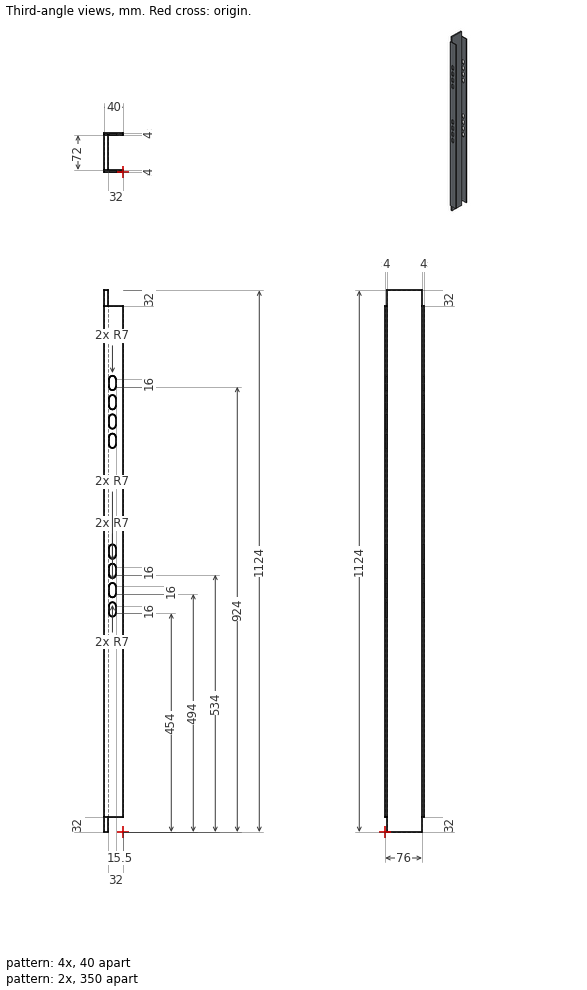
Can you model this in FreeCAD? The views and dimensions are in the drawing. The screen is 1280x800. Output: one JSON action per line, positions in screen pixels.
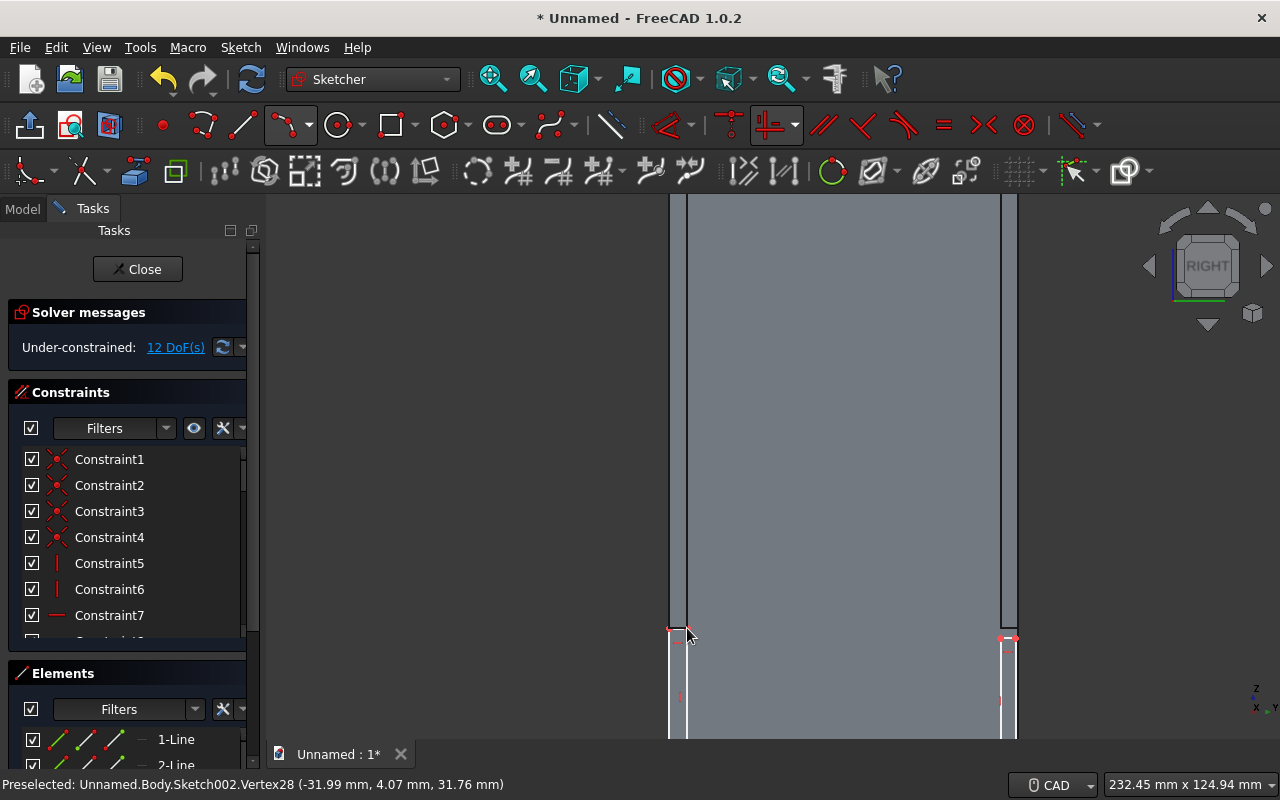
{"action": "left_click", "coordinate": [666, 126]}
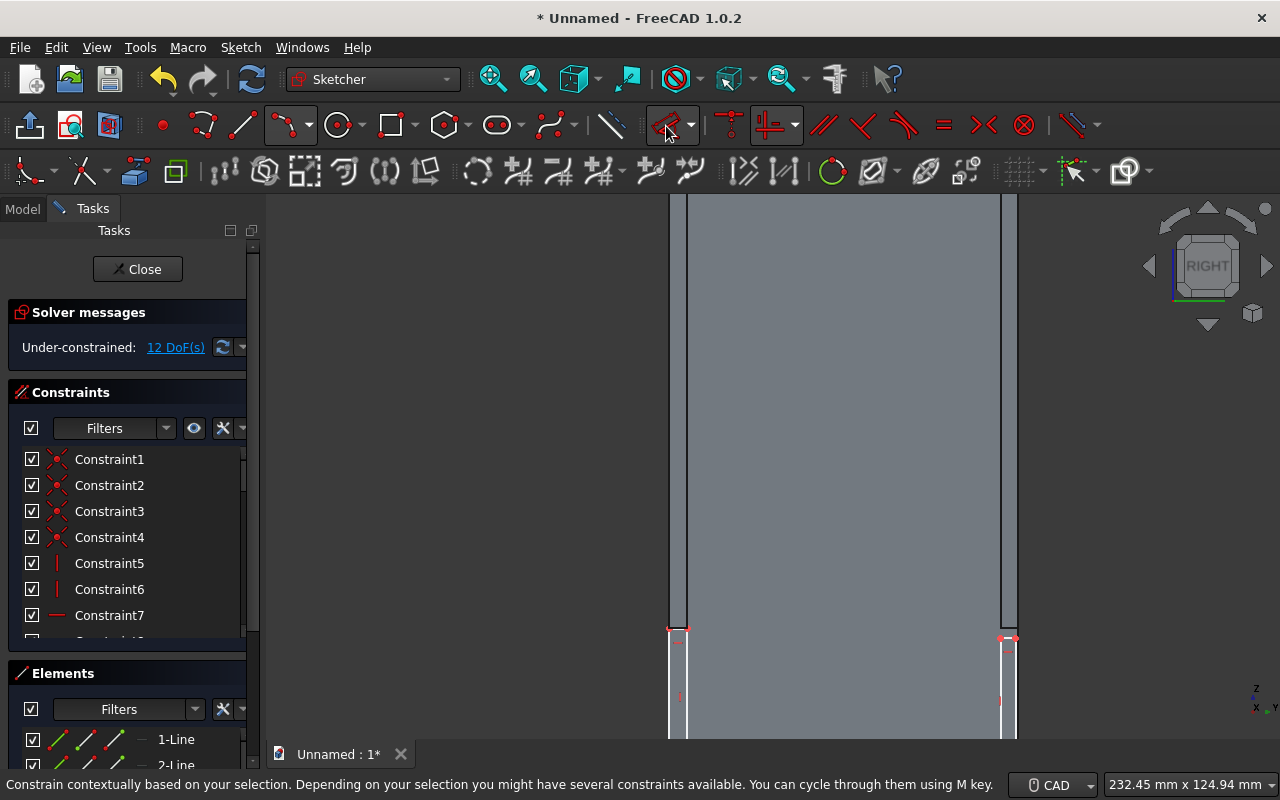
{"action": "scroll", "coordinate": [693, 639], "scroll_direction": "down", "scroll_amount": 13}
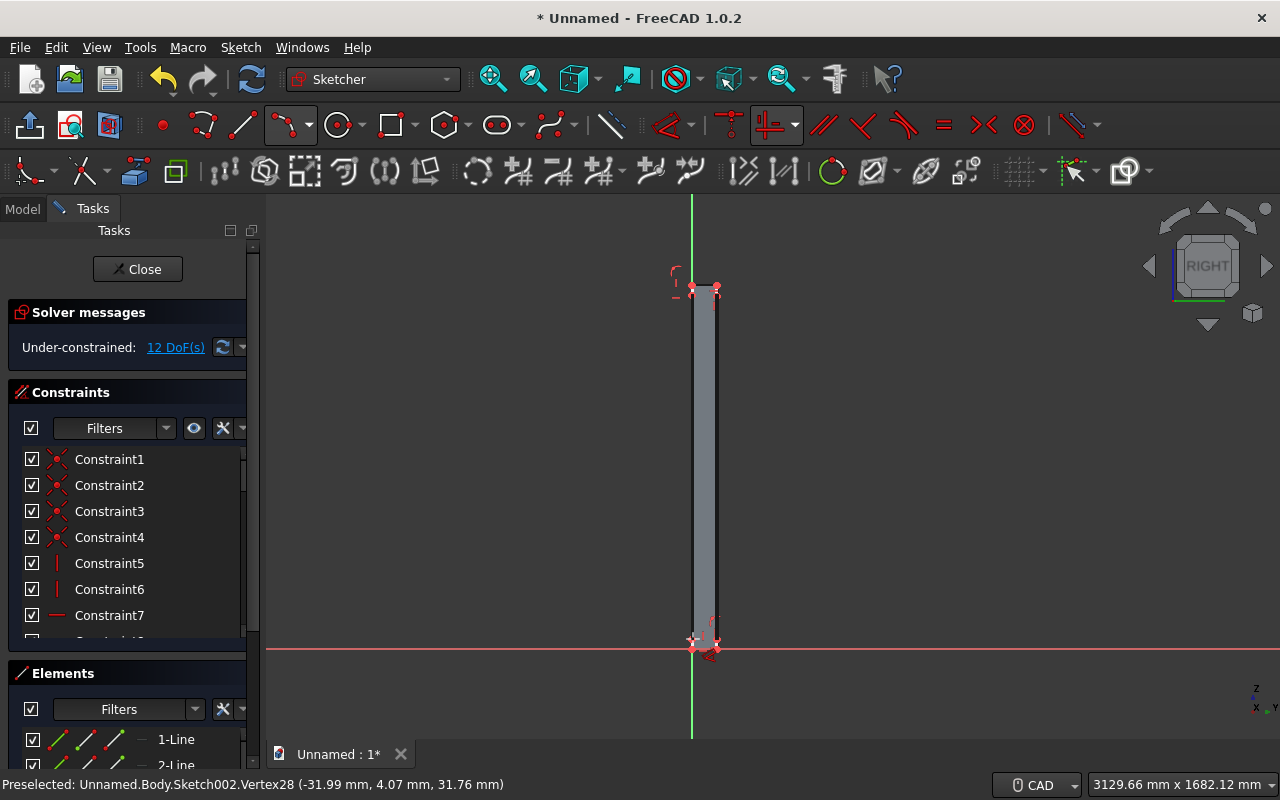
{"action": "scroll", "coordinate": [717, 297], "scroll_direction": "up", "scroll_amount": 18}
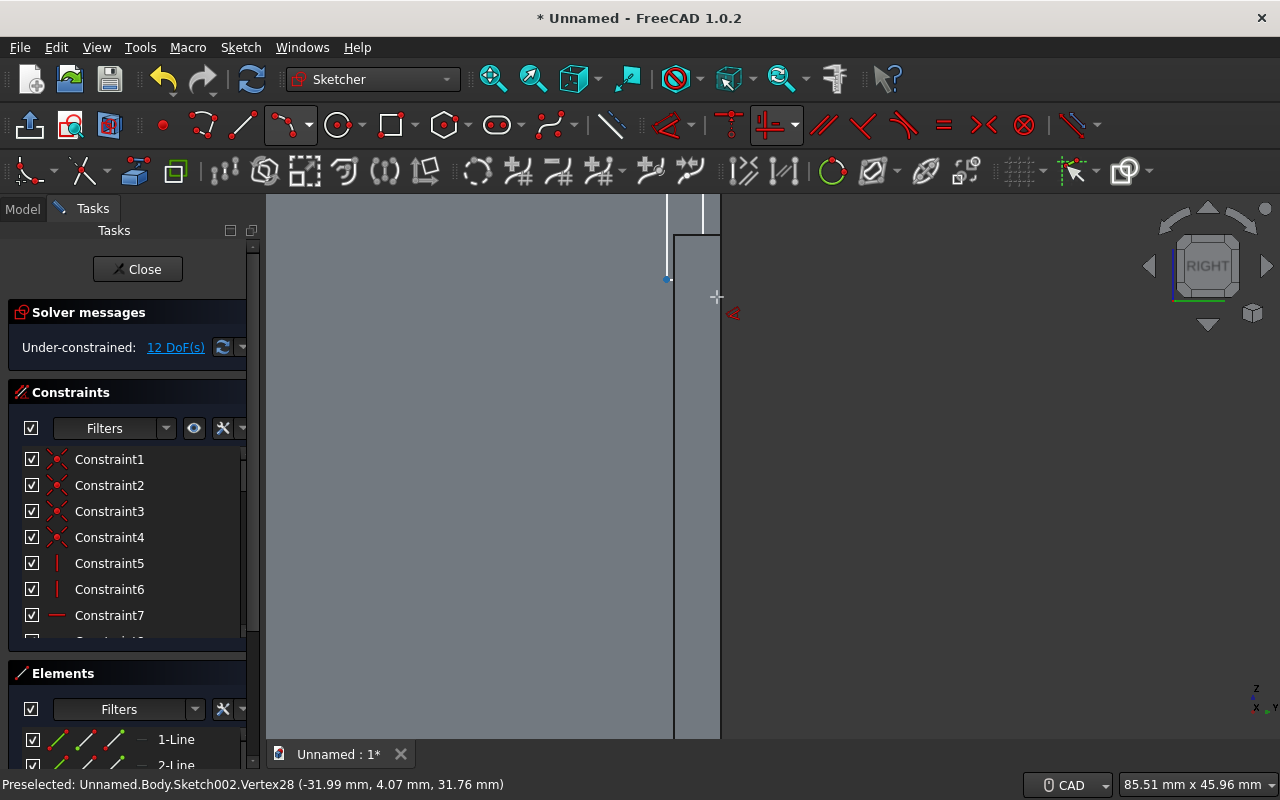
{"action": "left_click", "coordinate": [685, 280]}
{"action": "left_click", "coordinate": [685, 246]}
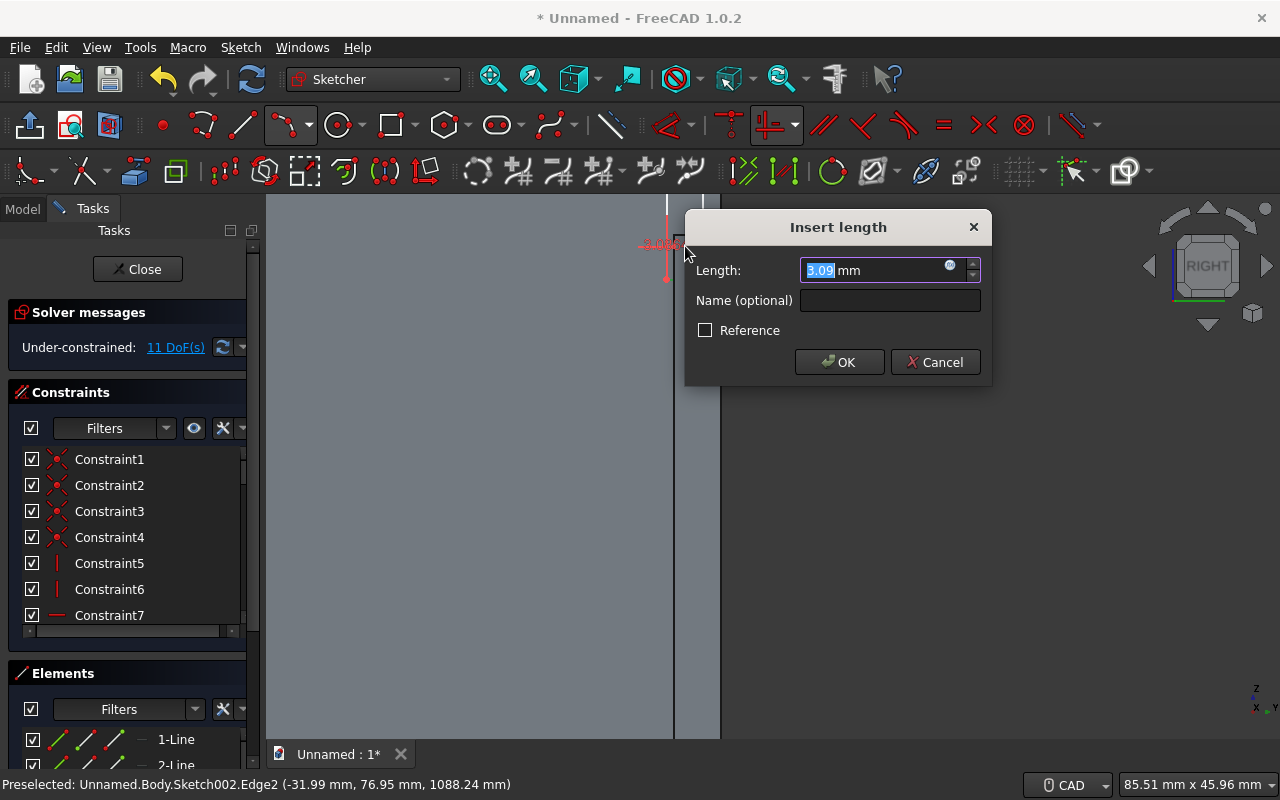
{"action": "type", "text": "4"}
{"action": "key", "text": "Return"}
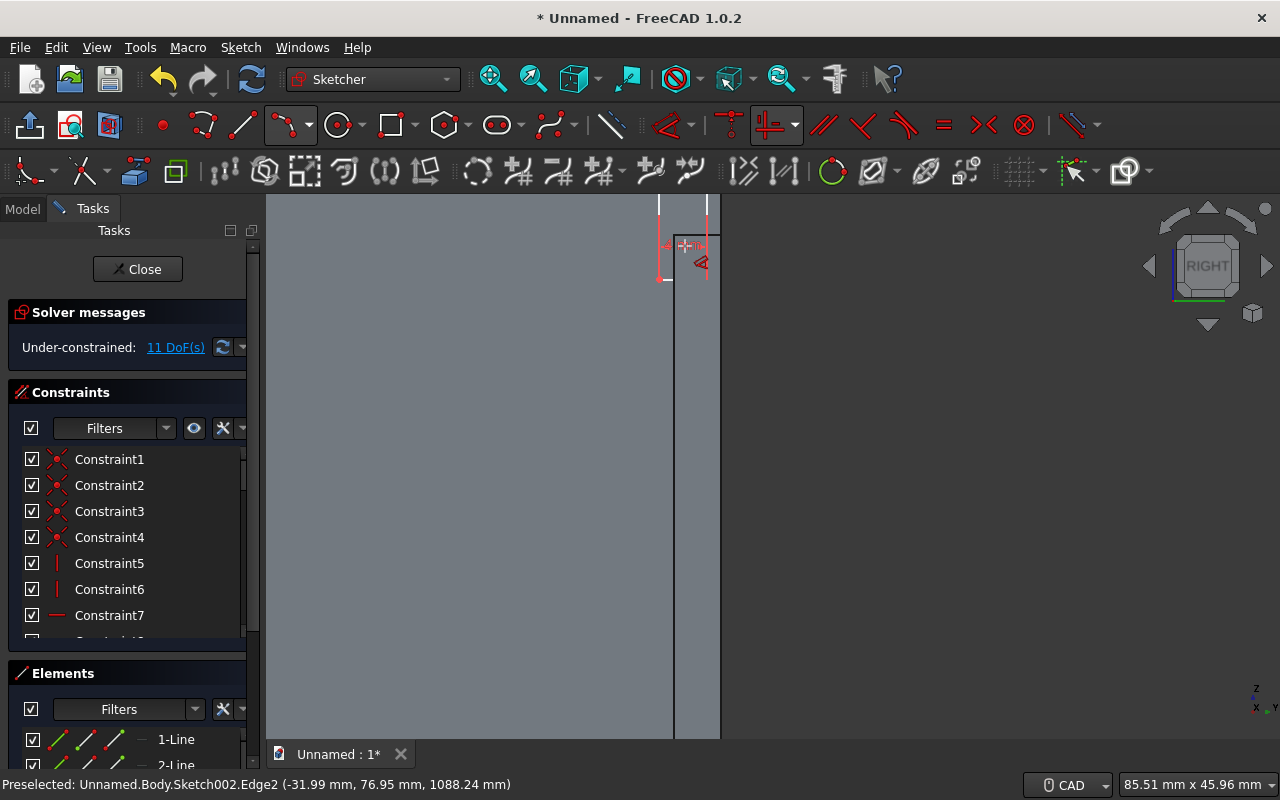
{"action": "scroll", "coordinate": [717, 296], "scroll_direction": "down", "scroll_amount": 18}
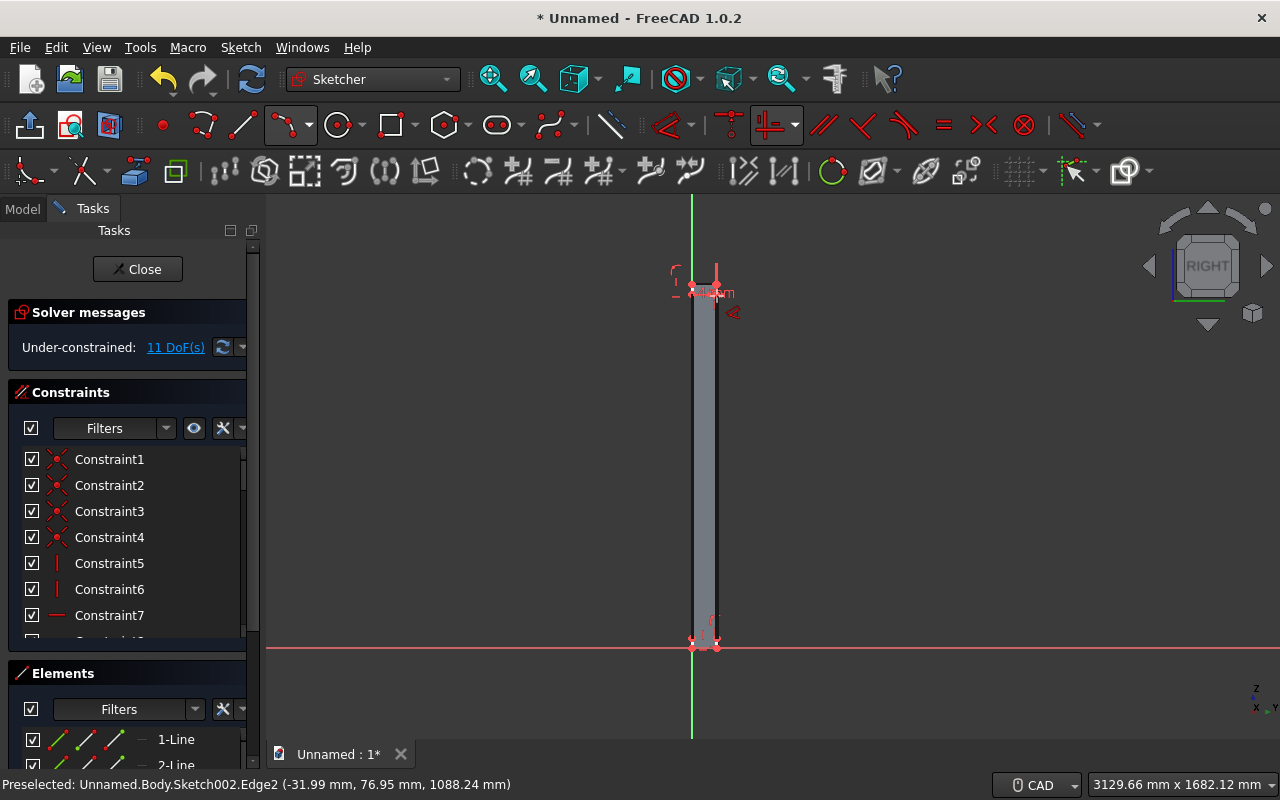
{"action": "scroll", "coordinate": [692, 295], "scroll_direction": "up", "scroll_amount": 18}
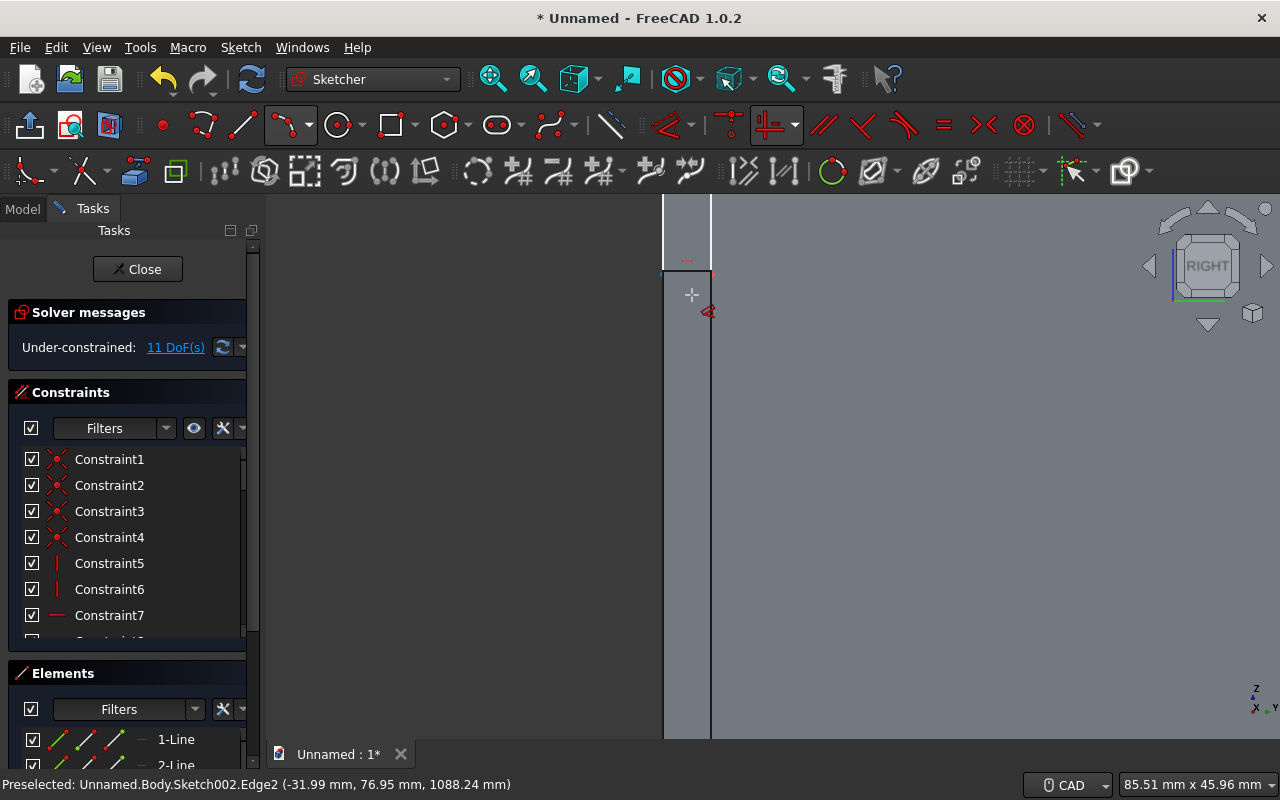
{"action": "left_click", "coordinate": [678, 274]}
{"action": "left_click", "coordinate": [687, 240]}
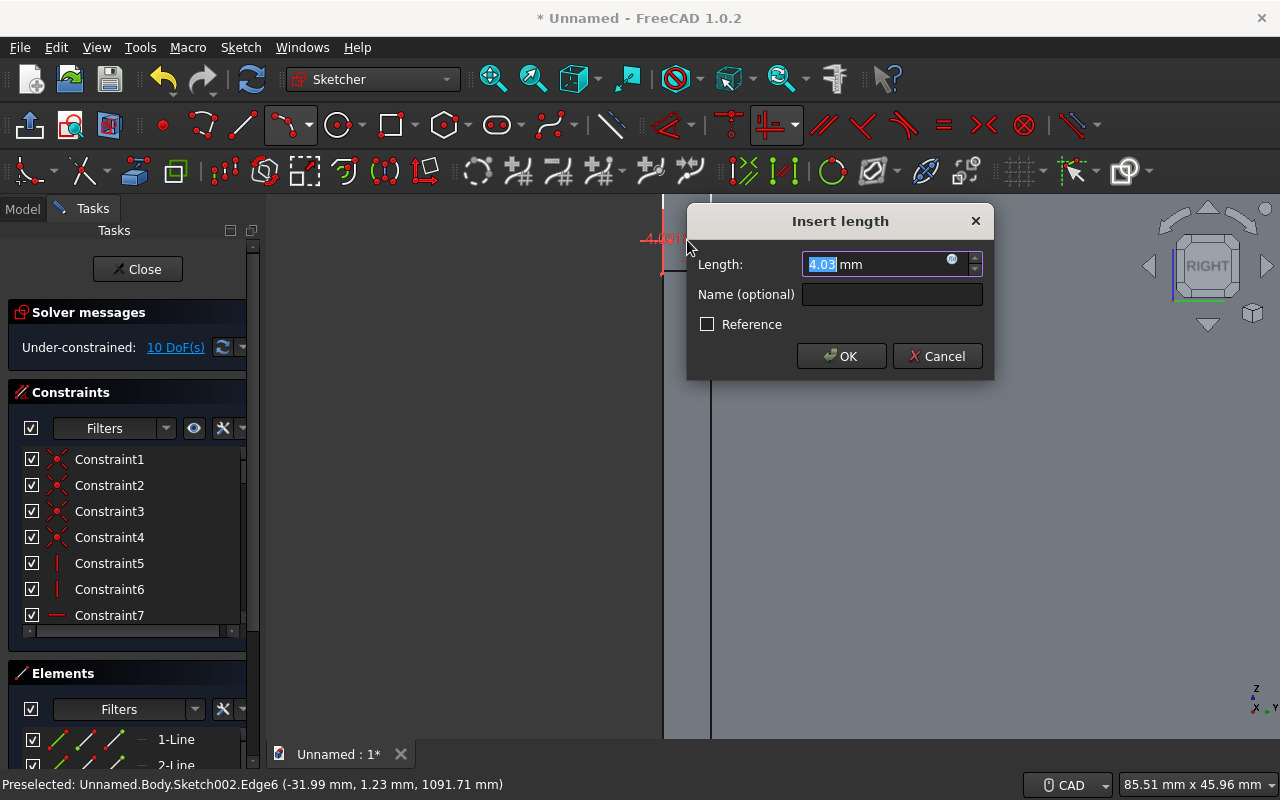
{"action": "type", "text": "4"}
{"action": "key", "text": "Return"}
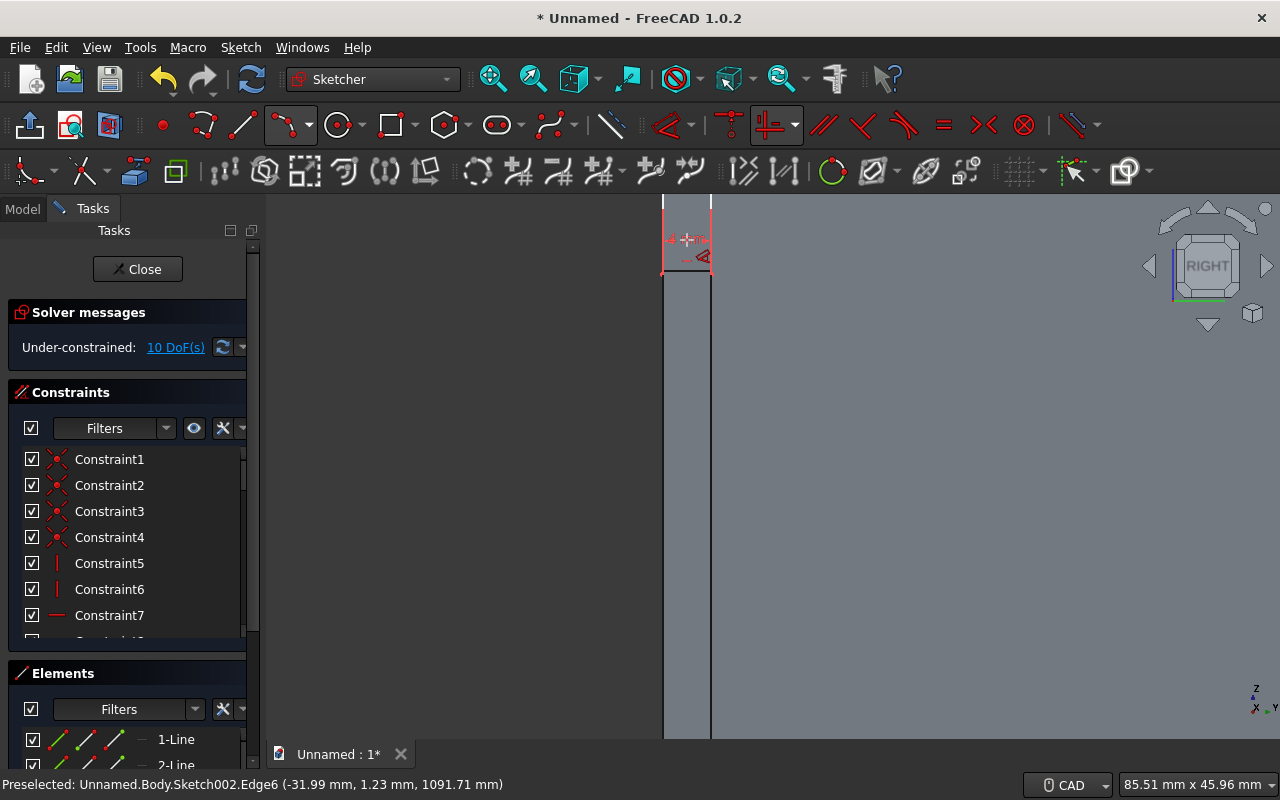
{"action": "scroll", "coordinate": [692, 295], "scroll_direction": "down", "scroll_amount": 18}